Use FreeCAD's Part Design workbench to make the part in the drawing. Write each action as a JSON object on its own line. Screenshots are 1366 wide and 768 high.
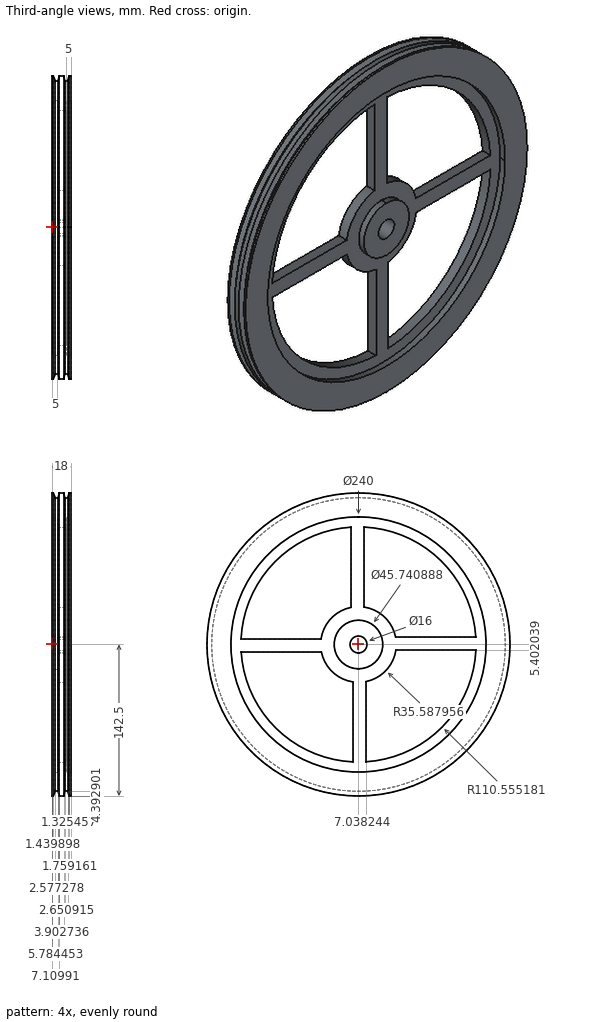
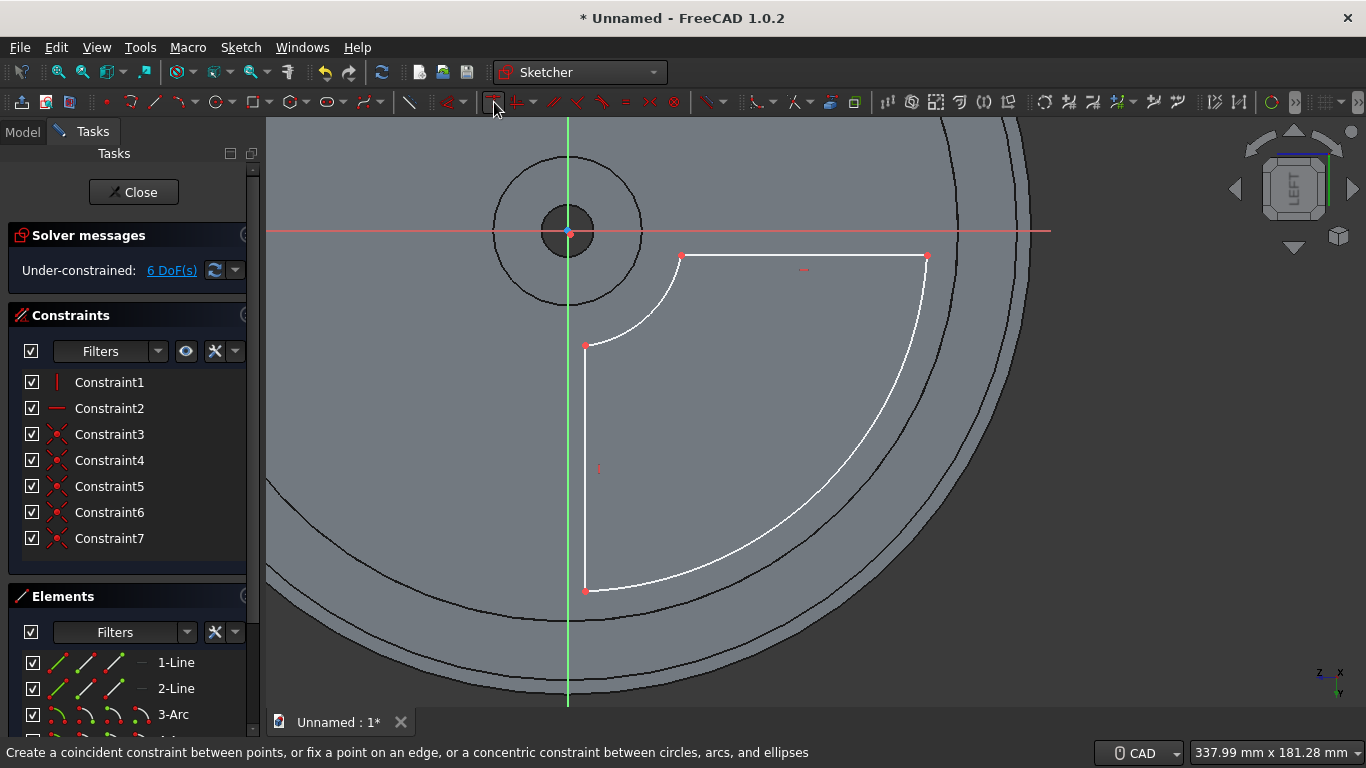
{"action": "left_click_drag", "start_coordinate": [558, 221], "coordinate": [581, 245]}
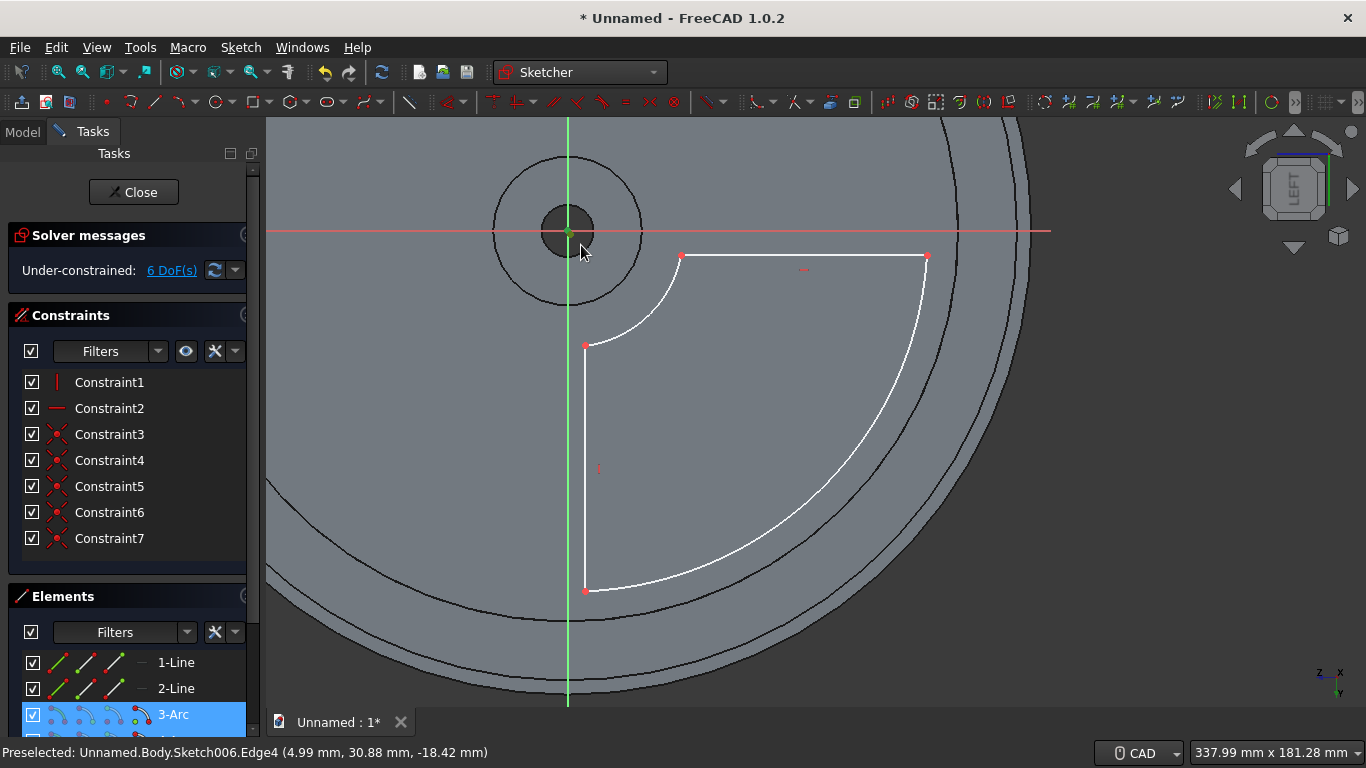
{"action": "left_click", "coordinate": [494, 102]}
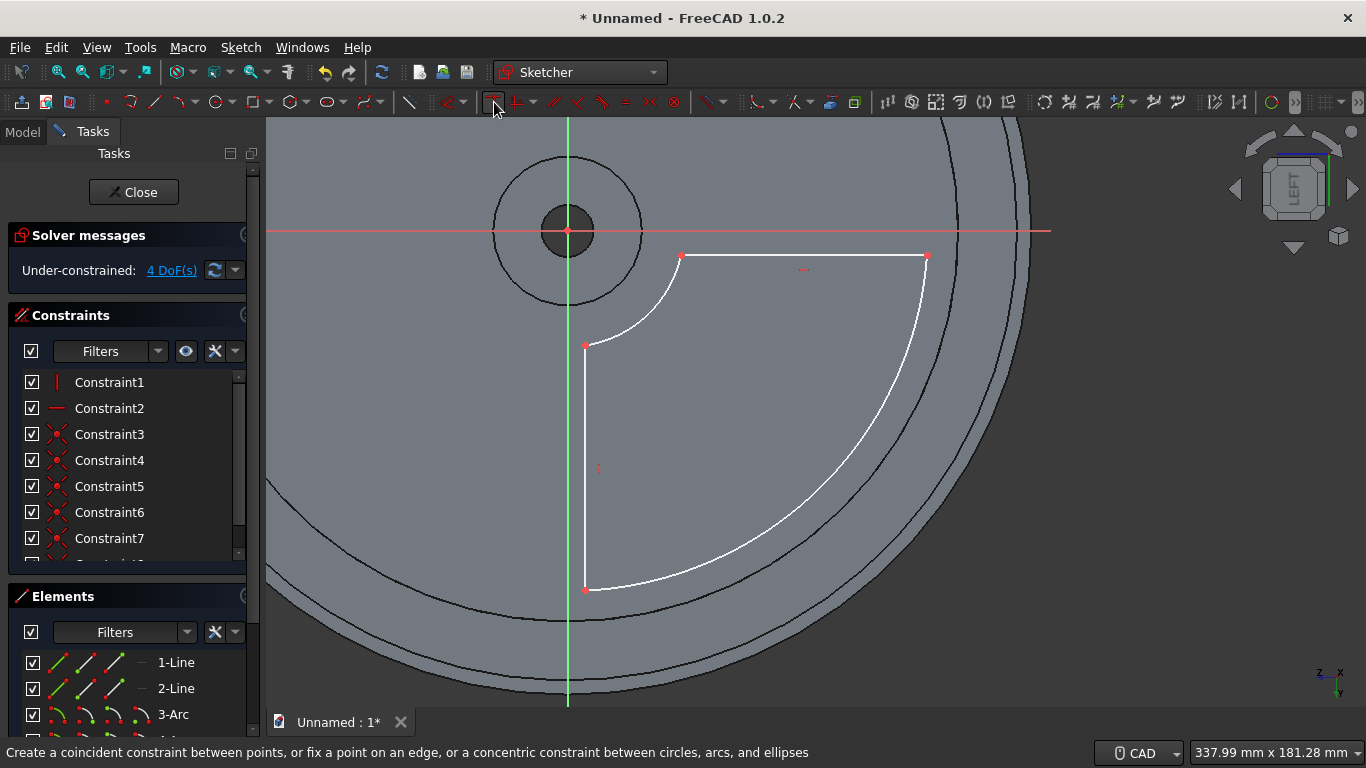
{"action": "key", "text": "d"}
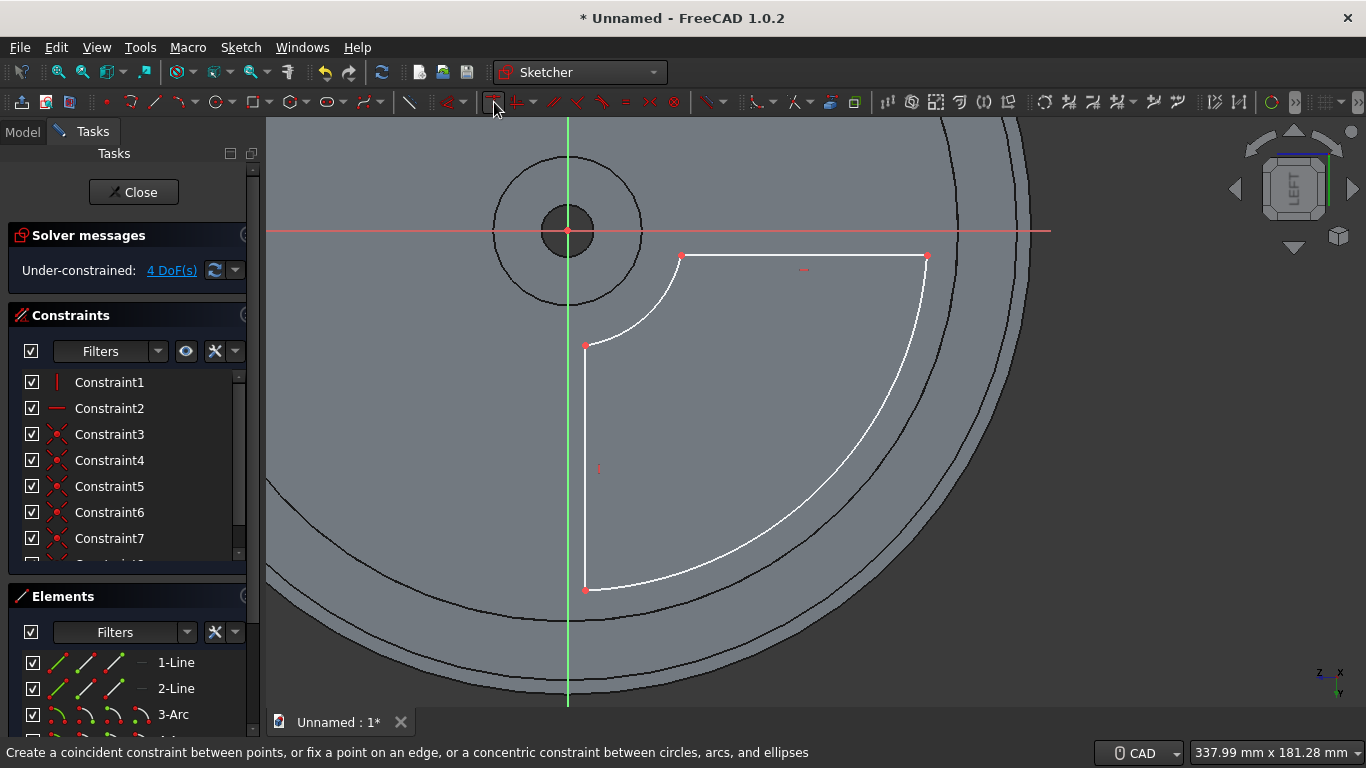
{"action": "left_click", "coordinate": [736, 550]}
{"action": "left_click", "coordinate": [751, 578]}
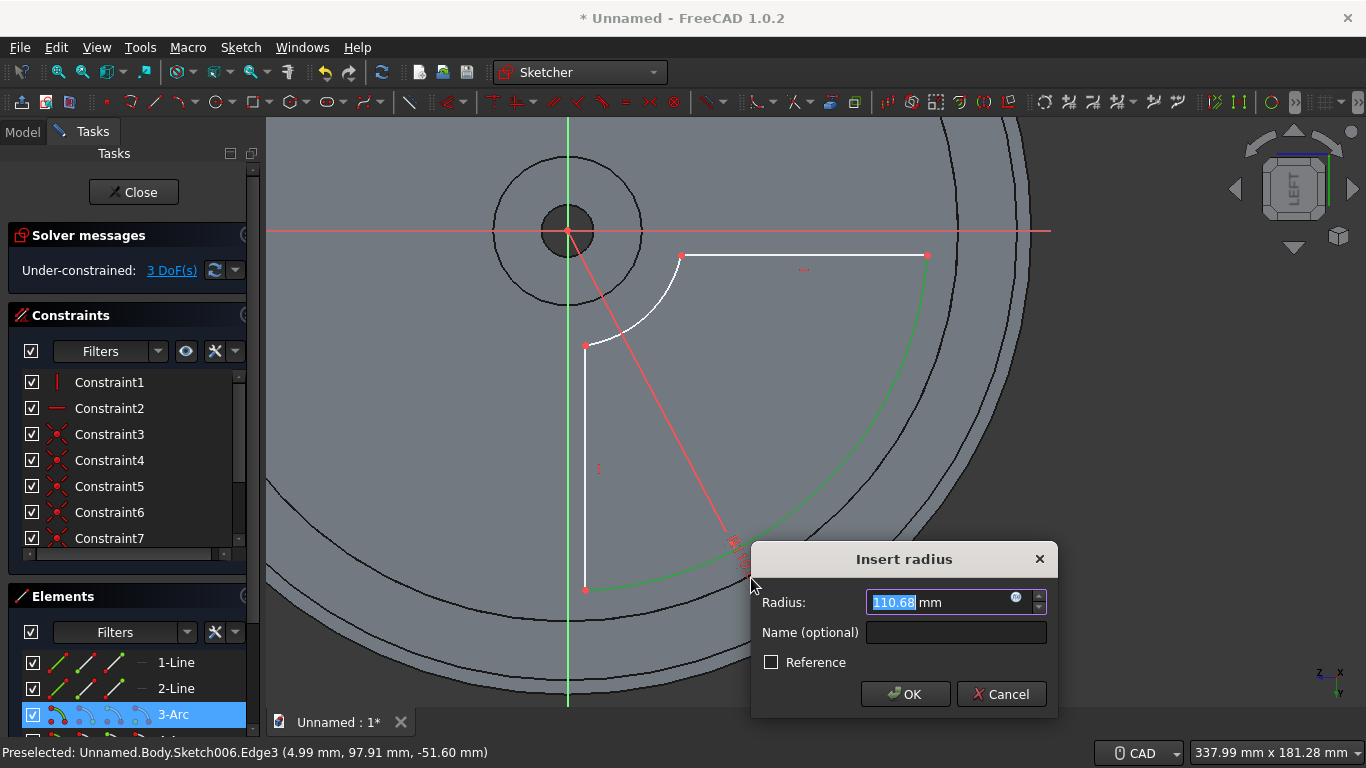
{"action": "type", "text": "110.555181"}
{"action": "key", "text": "Return"}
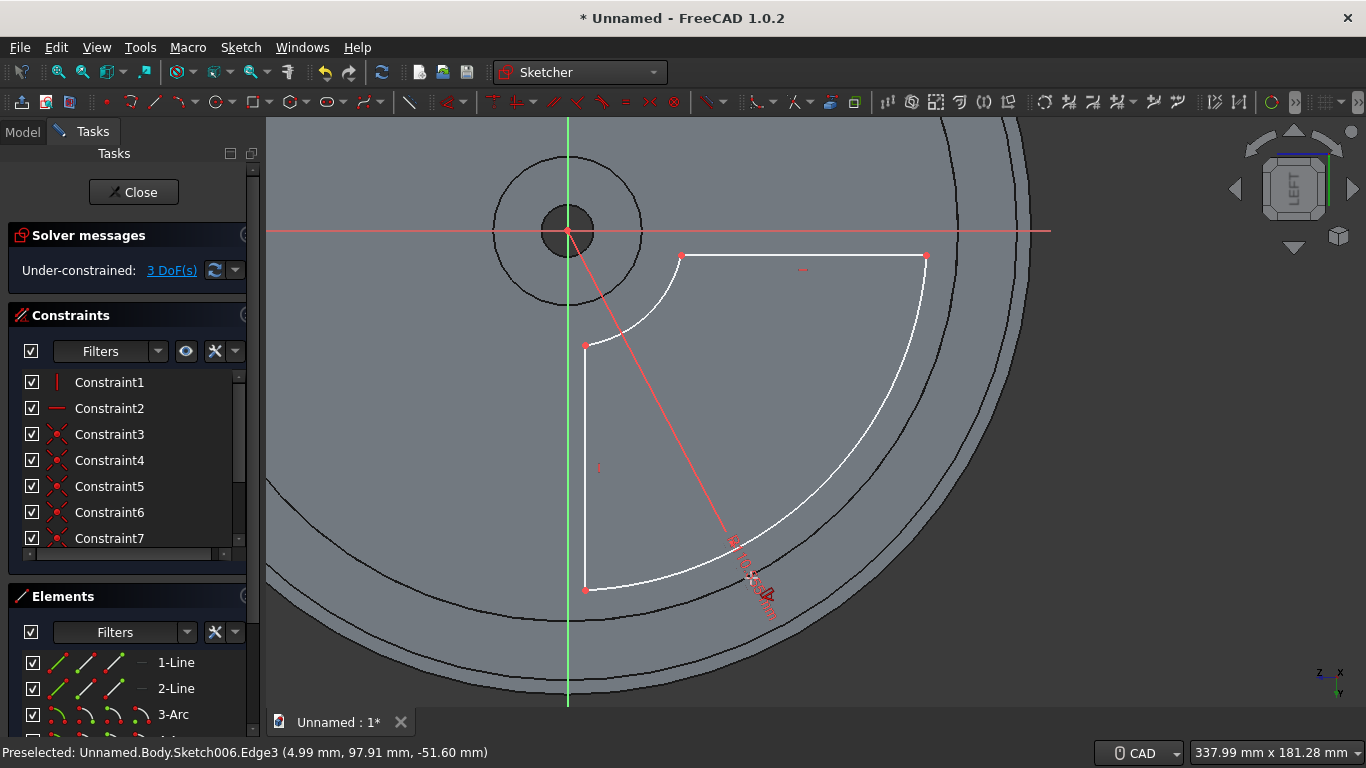
{"action": "left_click", "coordinate": [625, 332]}
{"action": "left_click", "coordinate": [641, 360]}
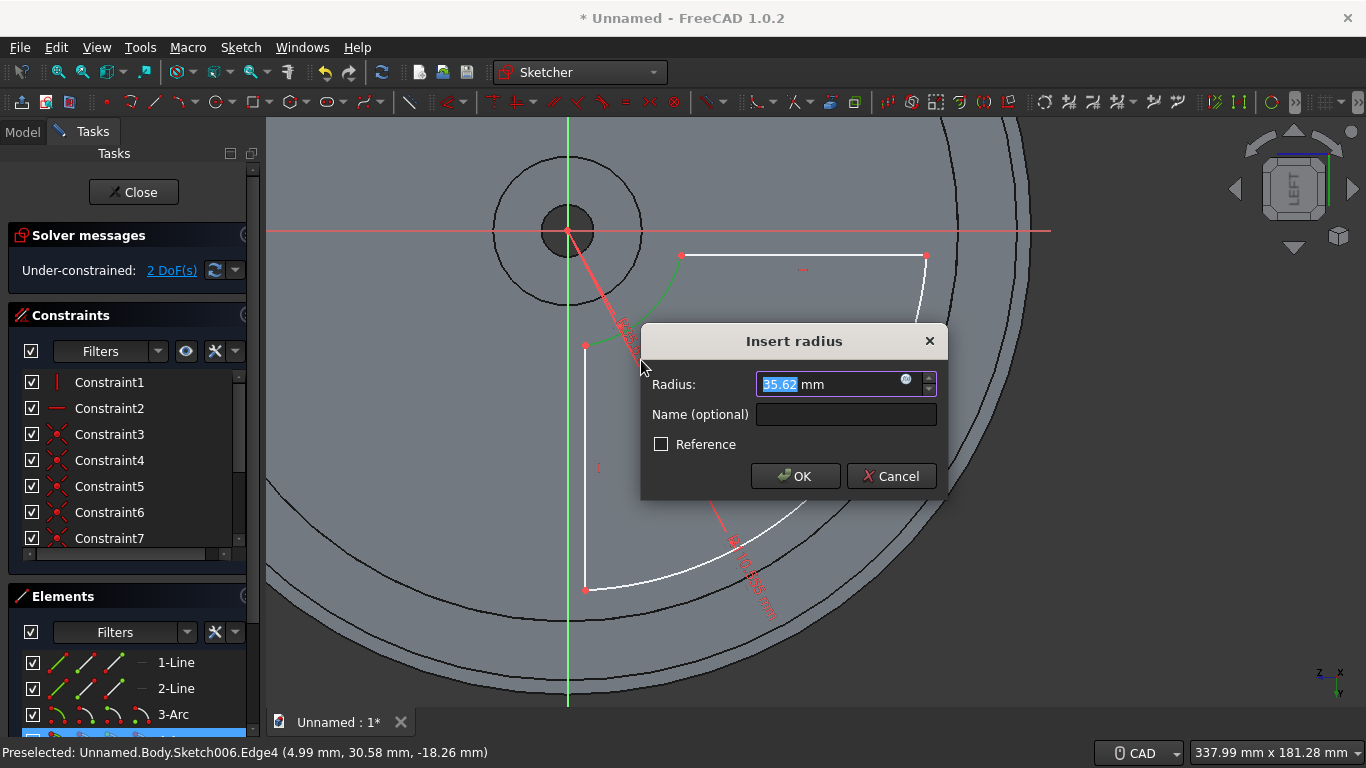
{"action": "type", "text": "35.587956"}
{"action": "key", "text": "Return"}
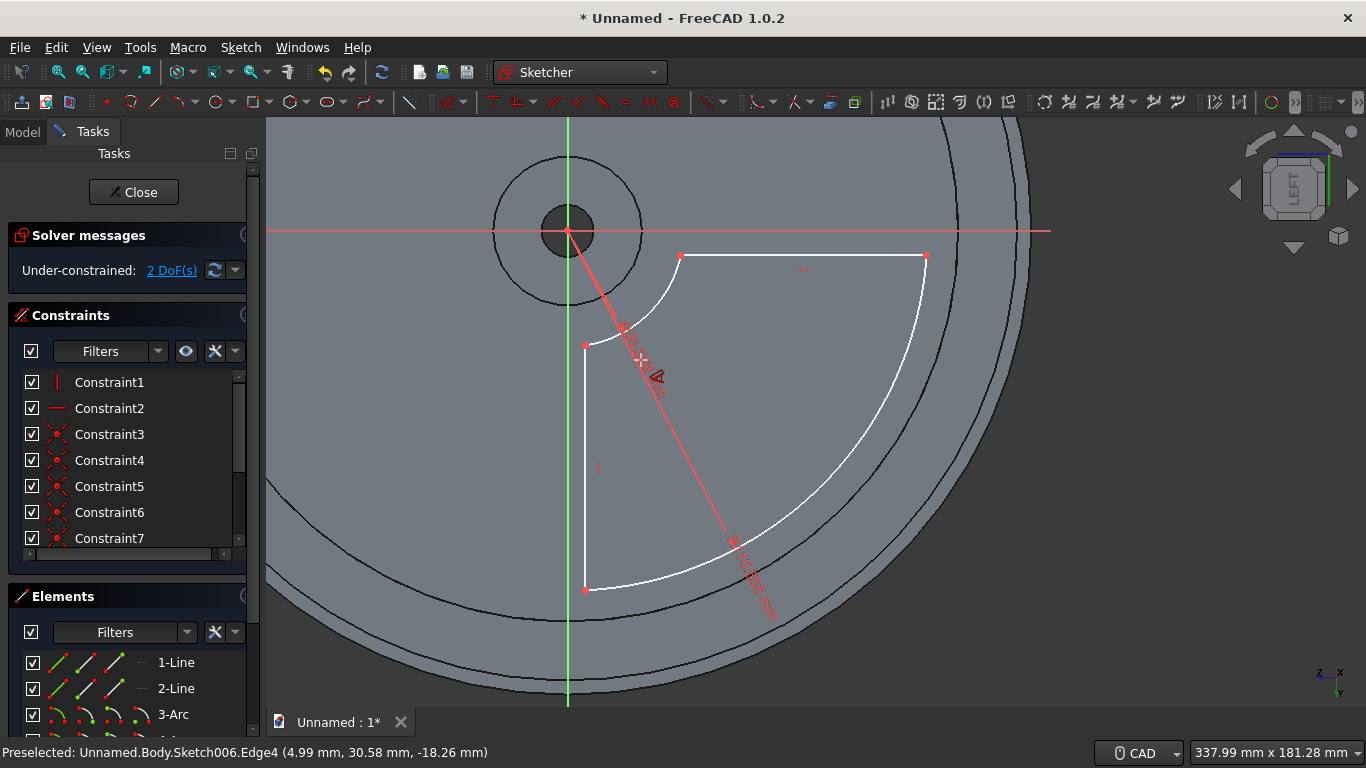
{"action": "scroll", "coordinate": [585, 345], "scroll_direction": "up", "scroll_amount": 5}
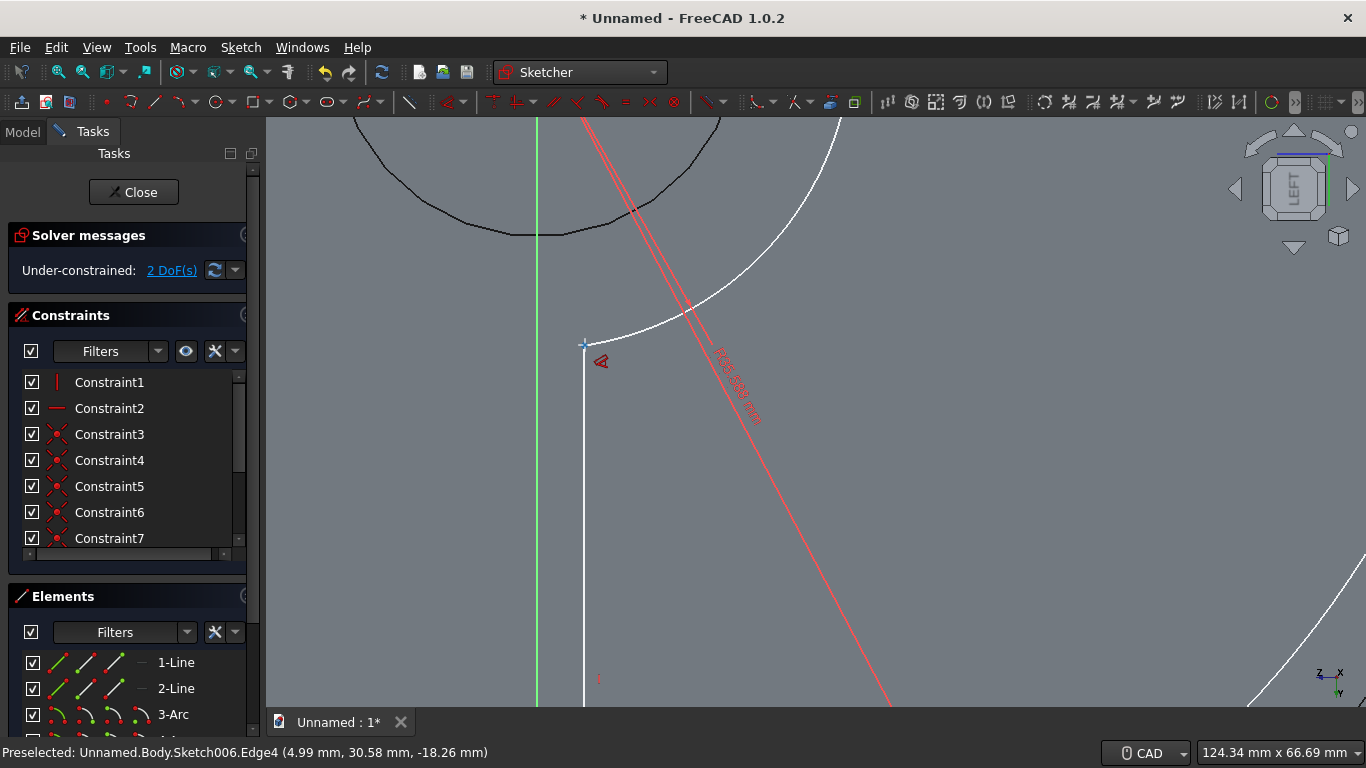
{"action": "left_click", "coordinate": [585, 346]}
{"action": "left_click", "coordinate": [561, 380]}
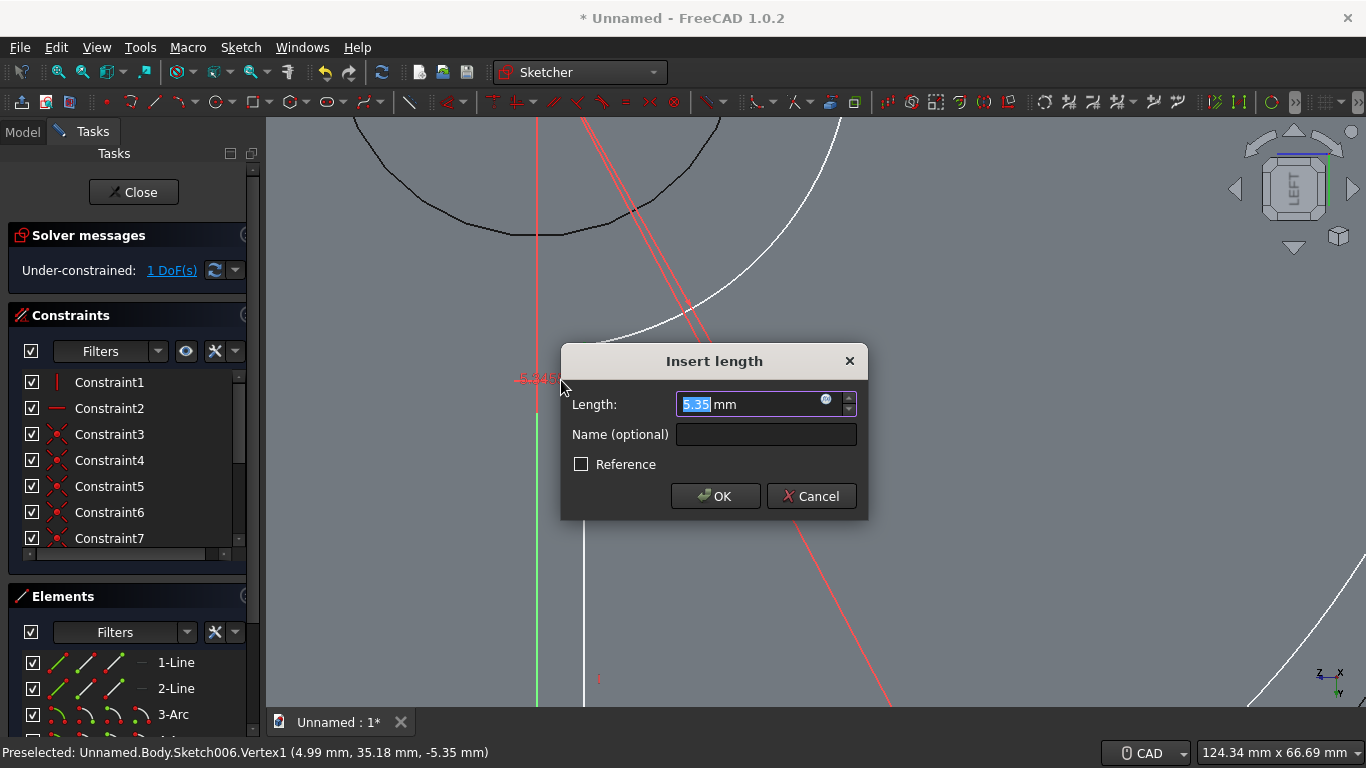
{"action": "type", "text": "5.402039"}
{"action": "key", "text": "Return"}